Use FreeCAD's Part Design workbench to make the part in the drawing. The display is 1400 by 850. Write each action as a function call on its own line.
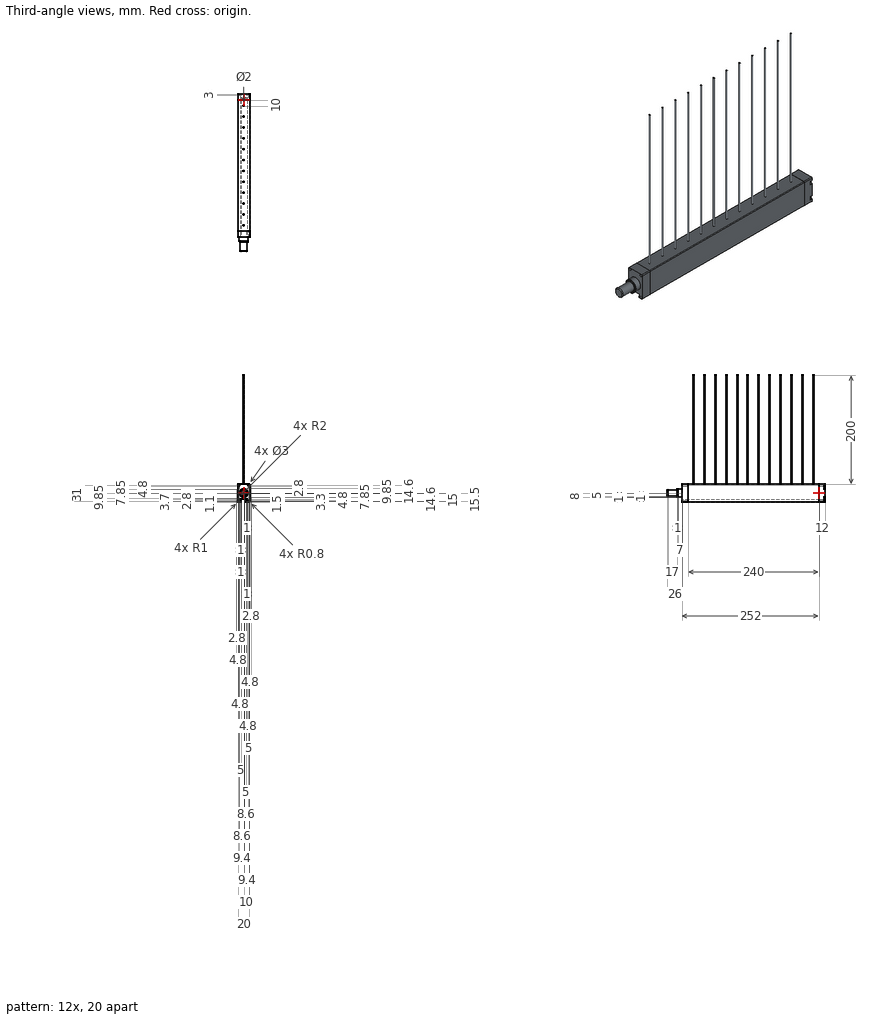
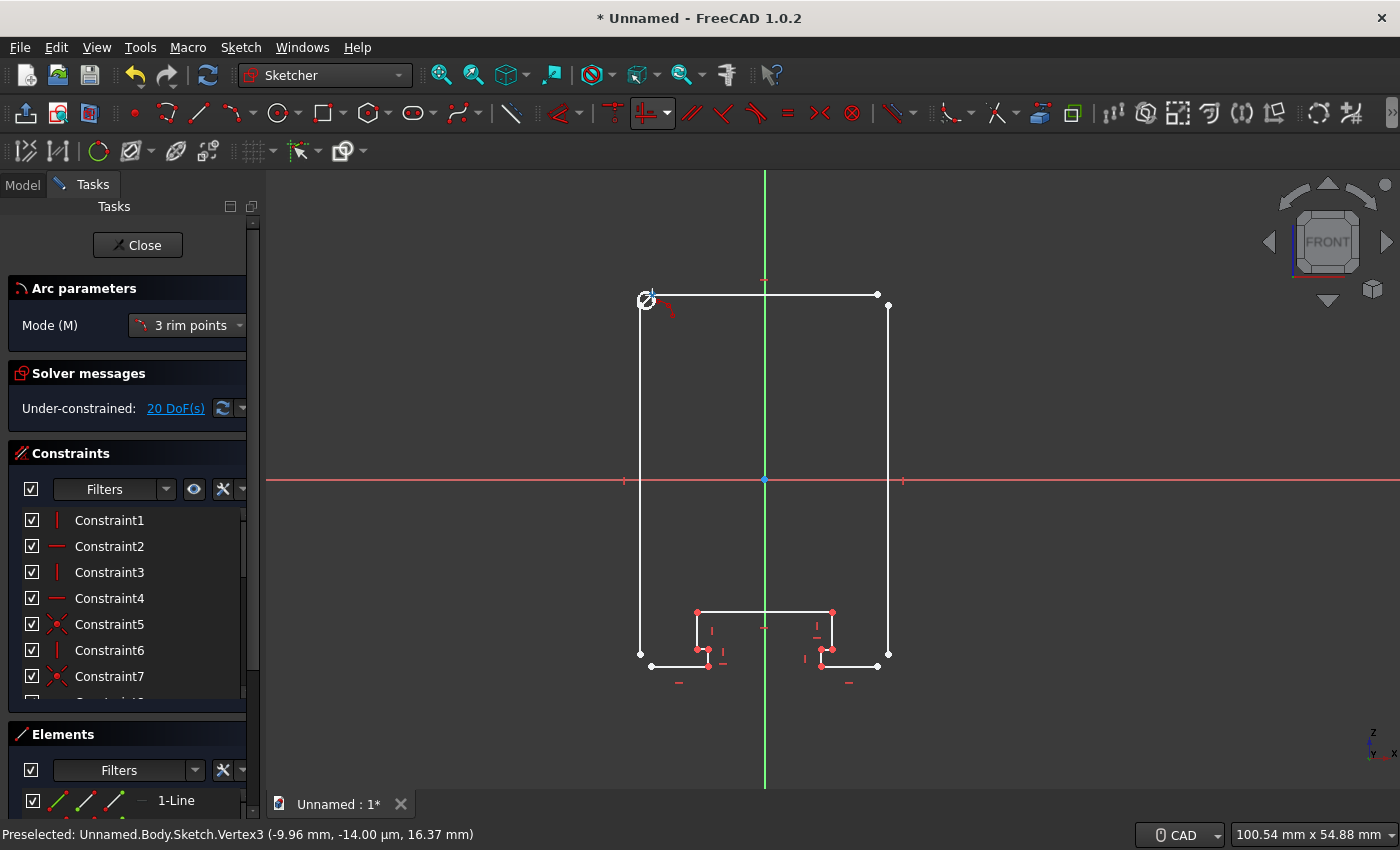
scroll(644, 297, up, 8)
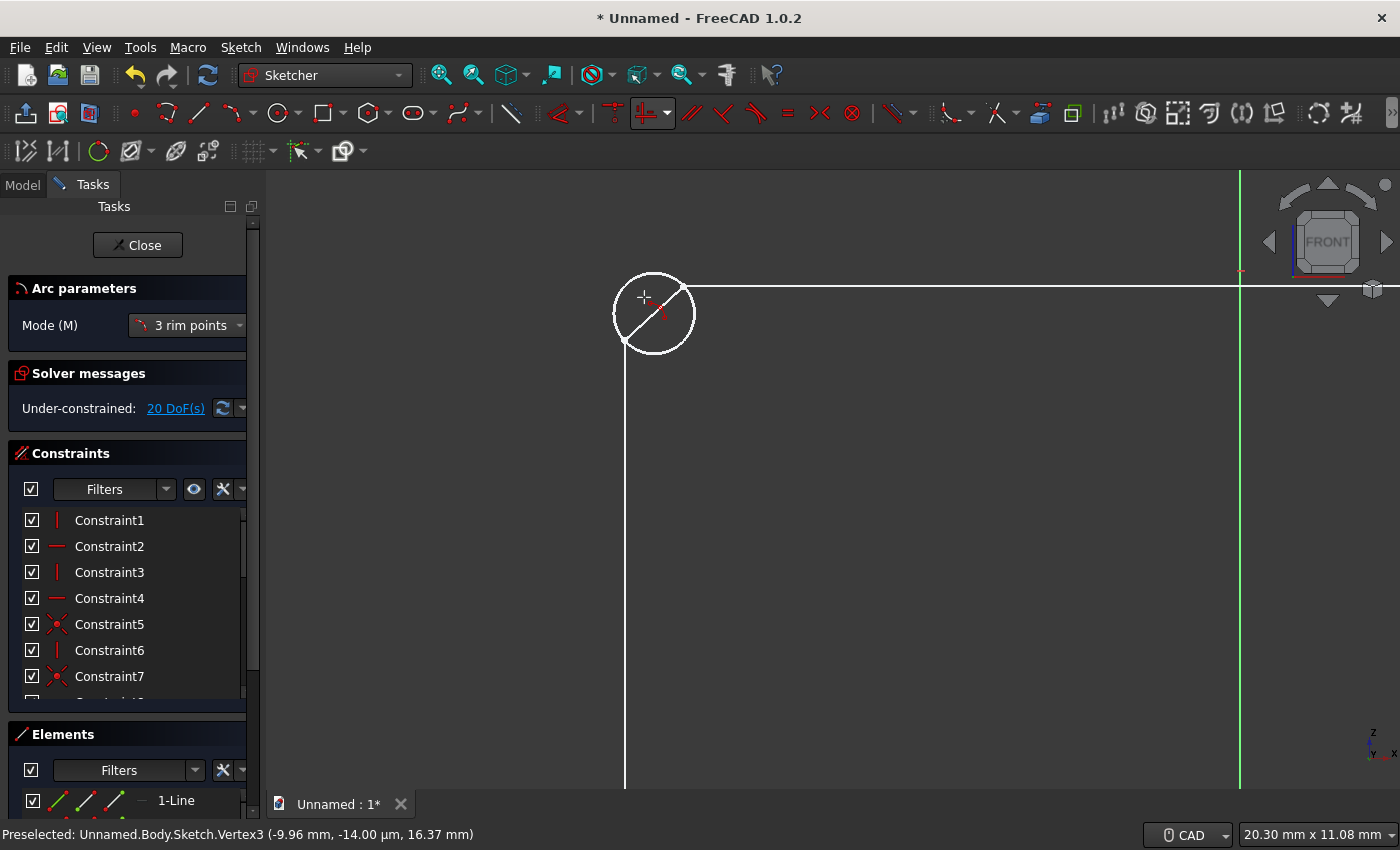
click(642, 296)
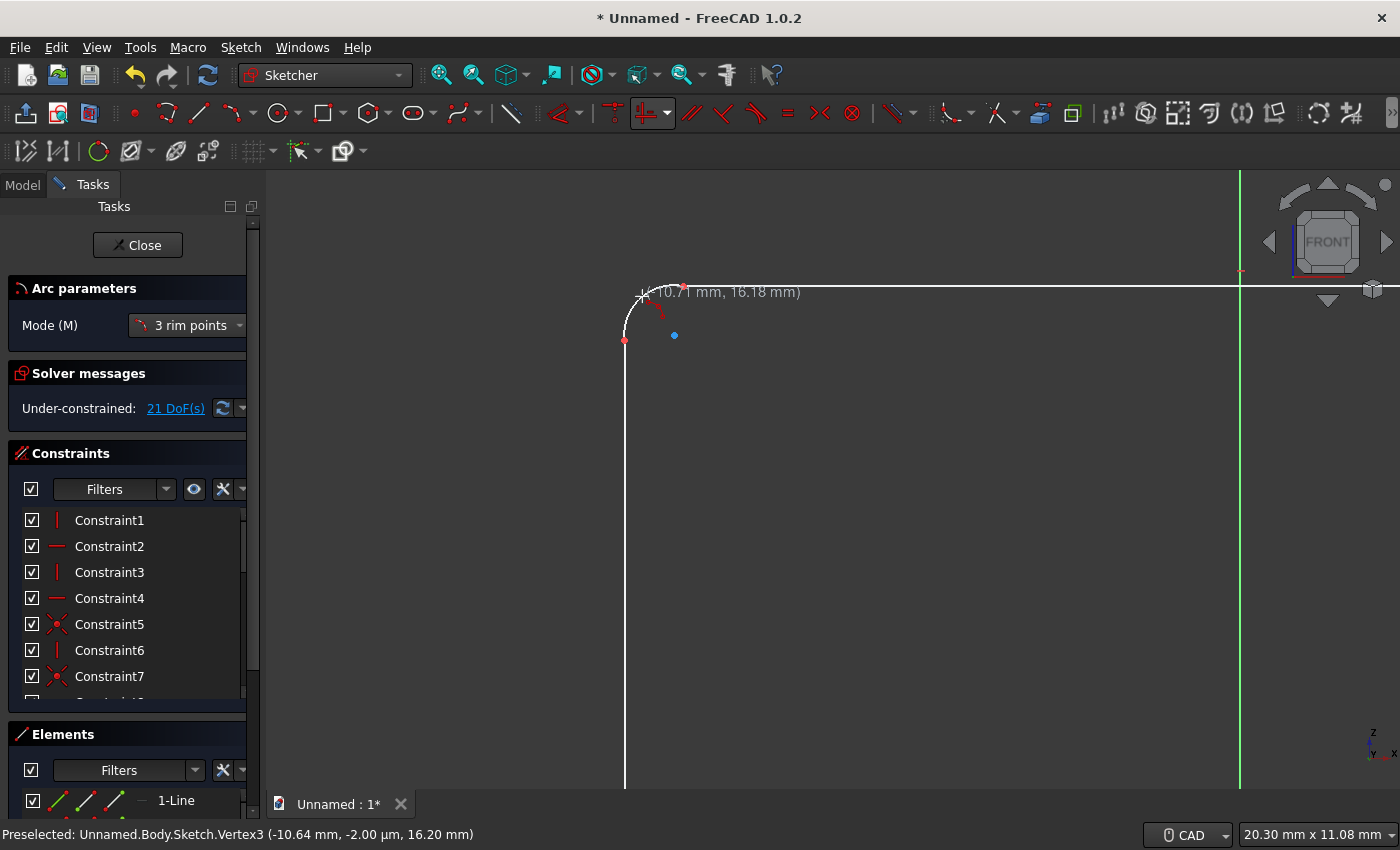
scroll(644, 297, down, 8)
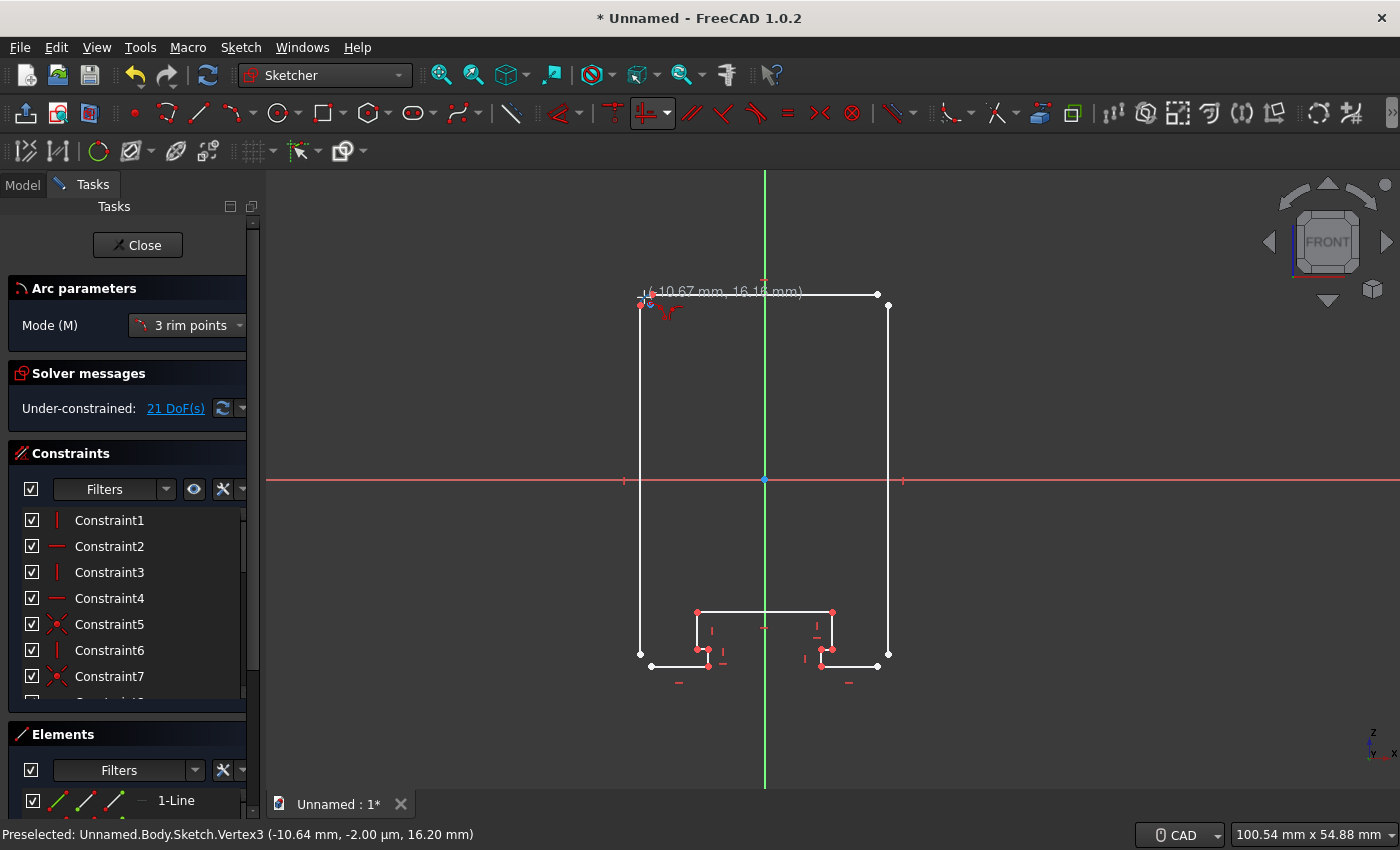
click(877, 295)
click(888, 306)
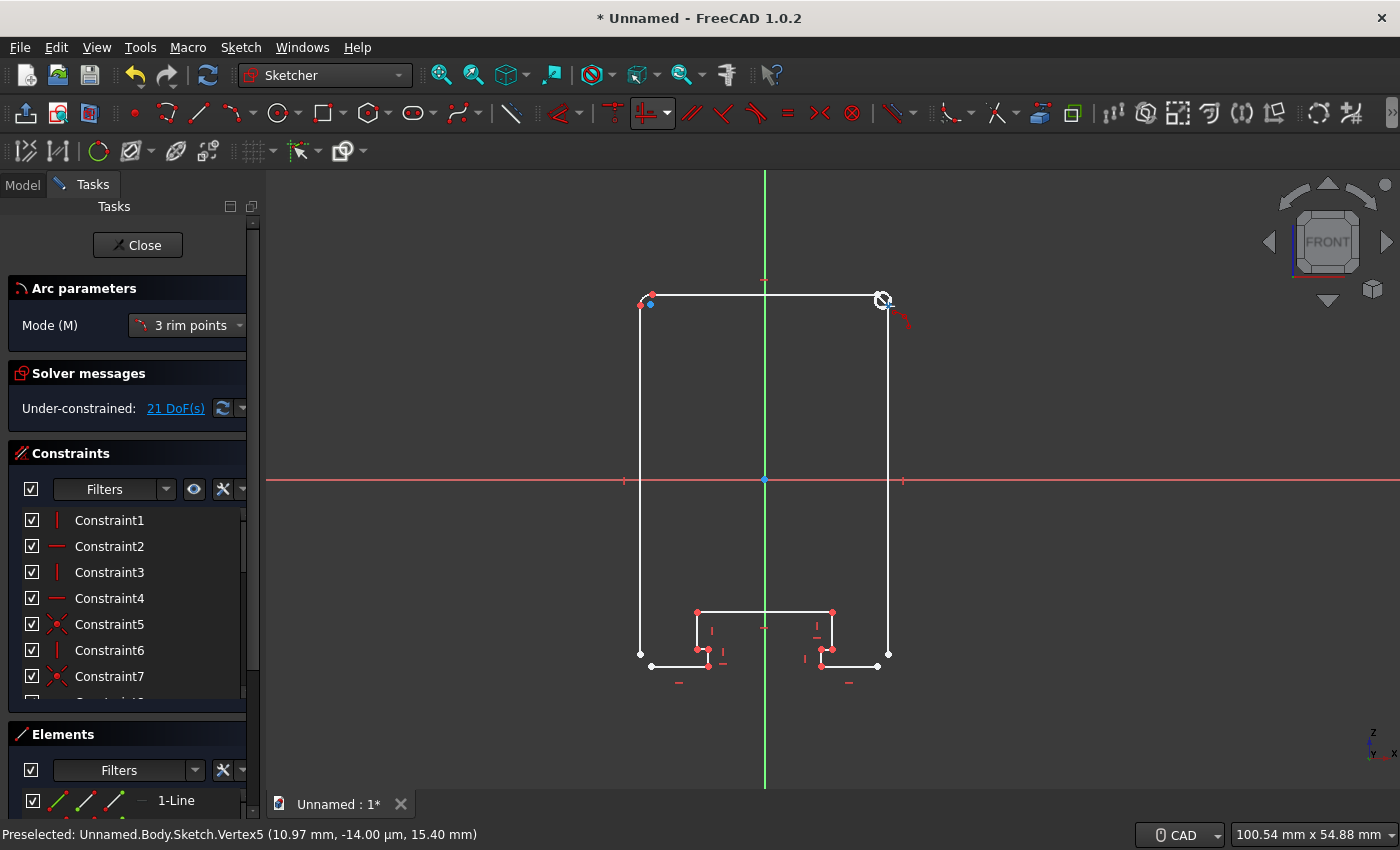
scroll(885, 297, up, 8)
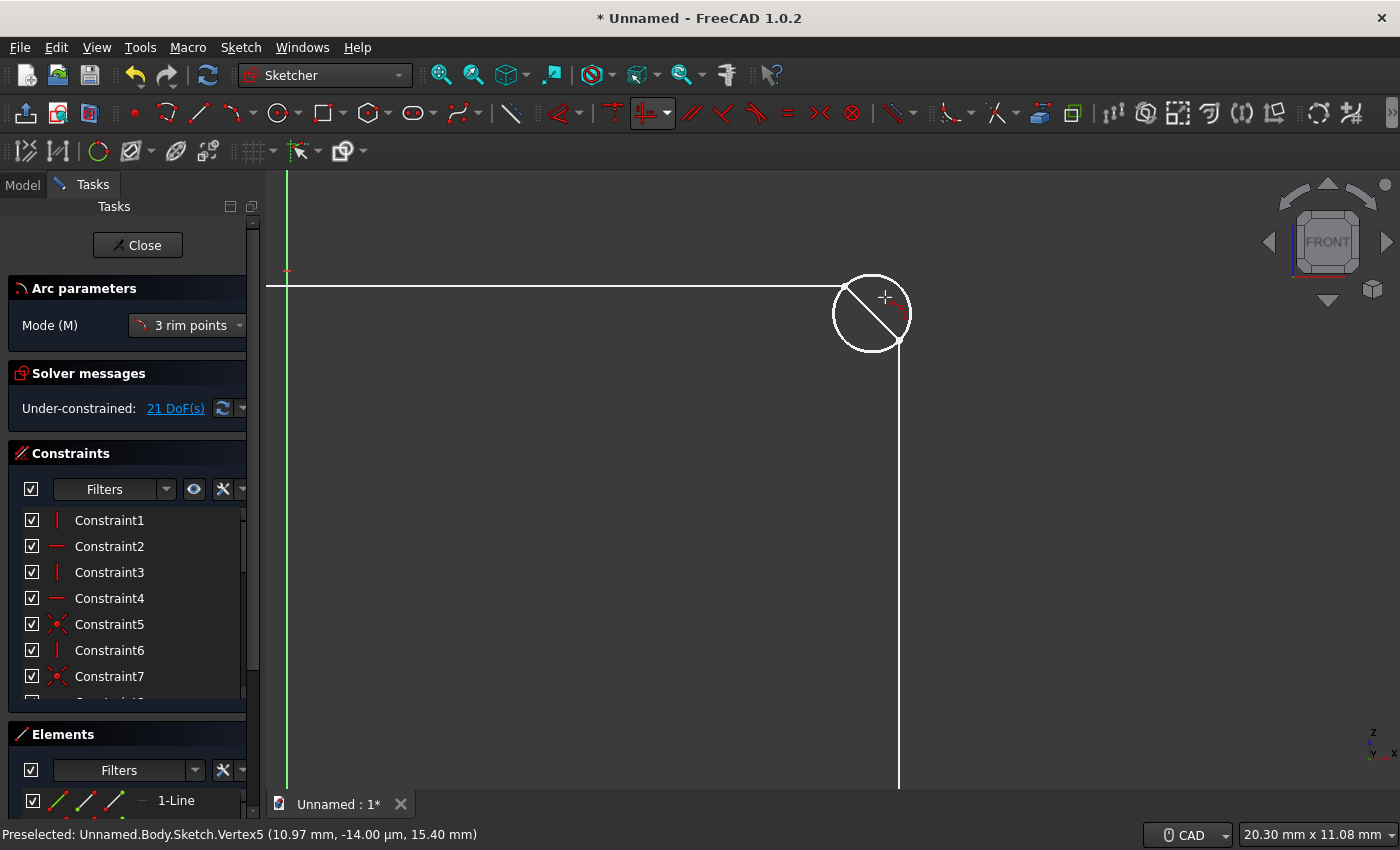
click(885, 296)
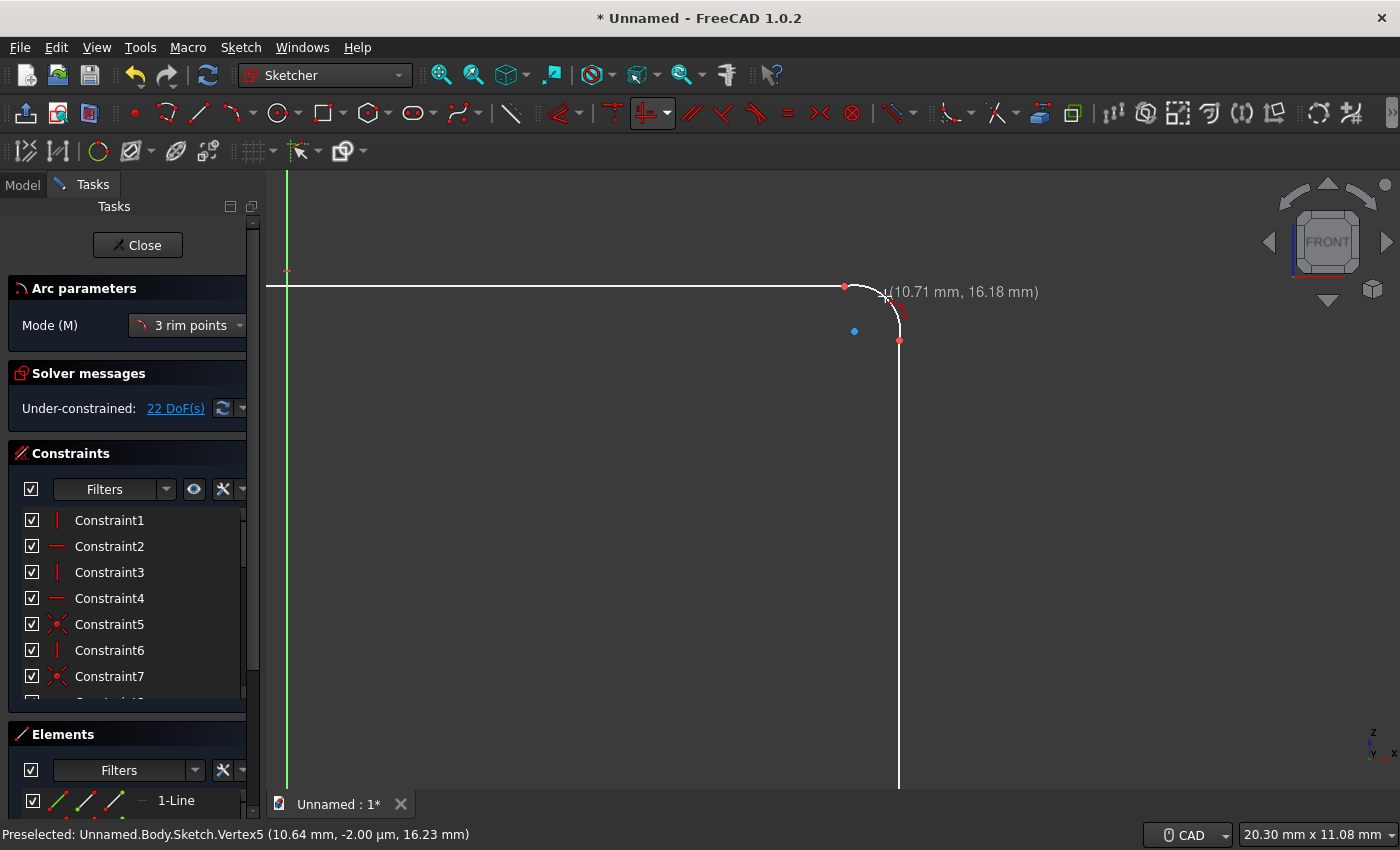
scroll(885, 297, down, 8)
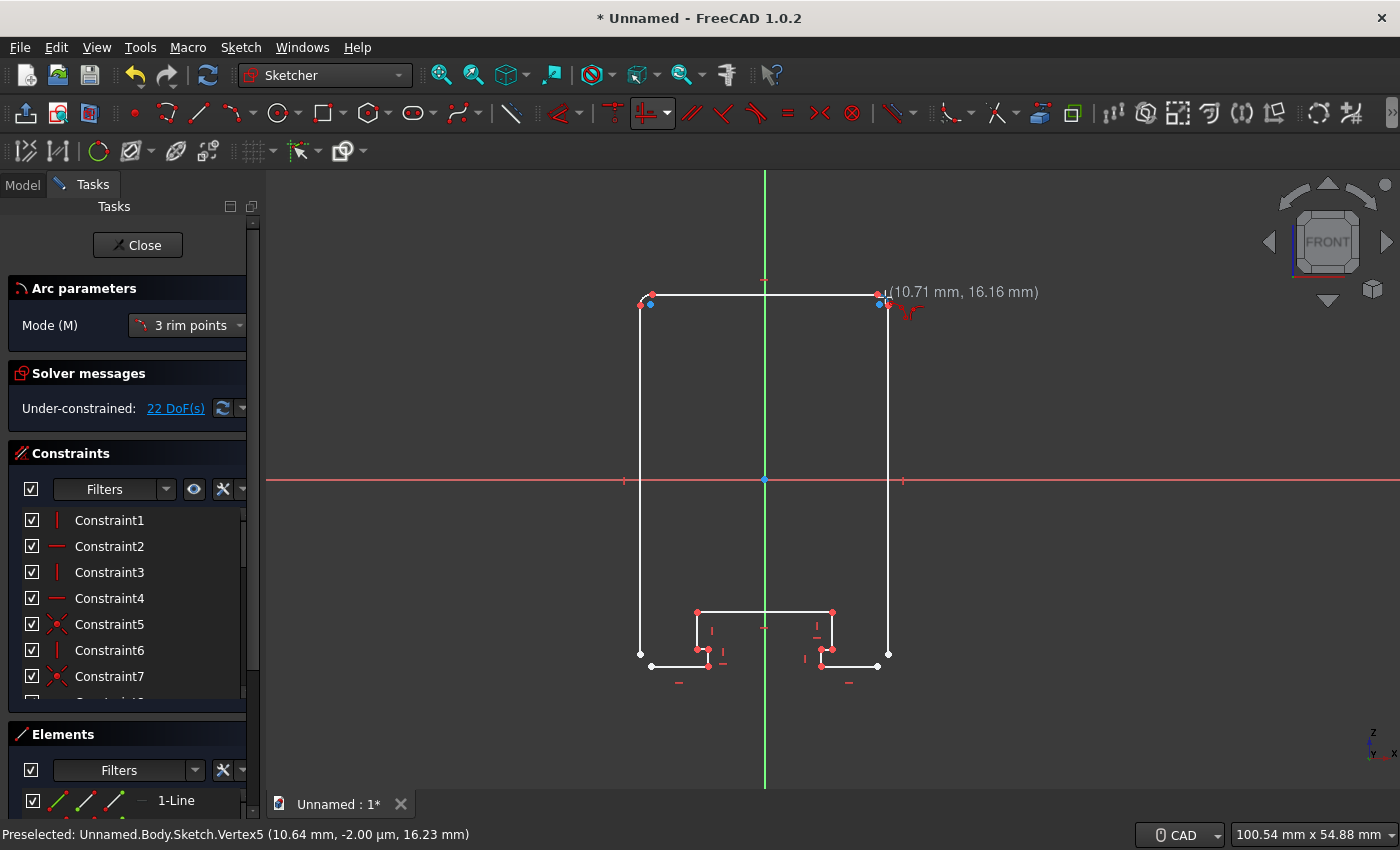
click(888, 655)
click(877, 667)